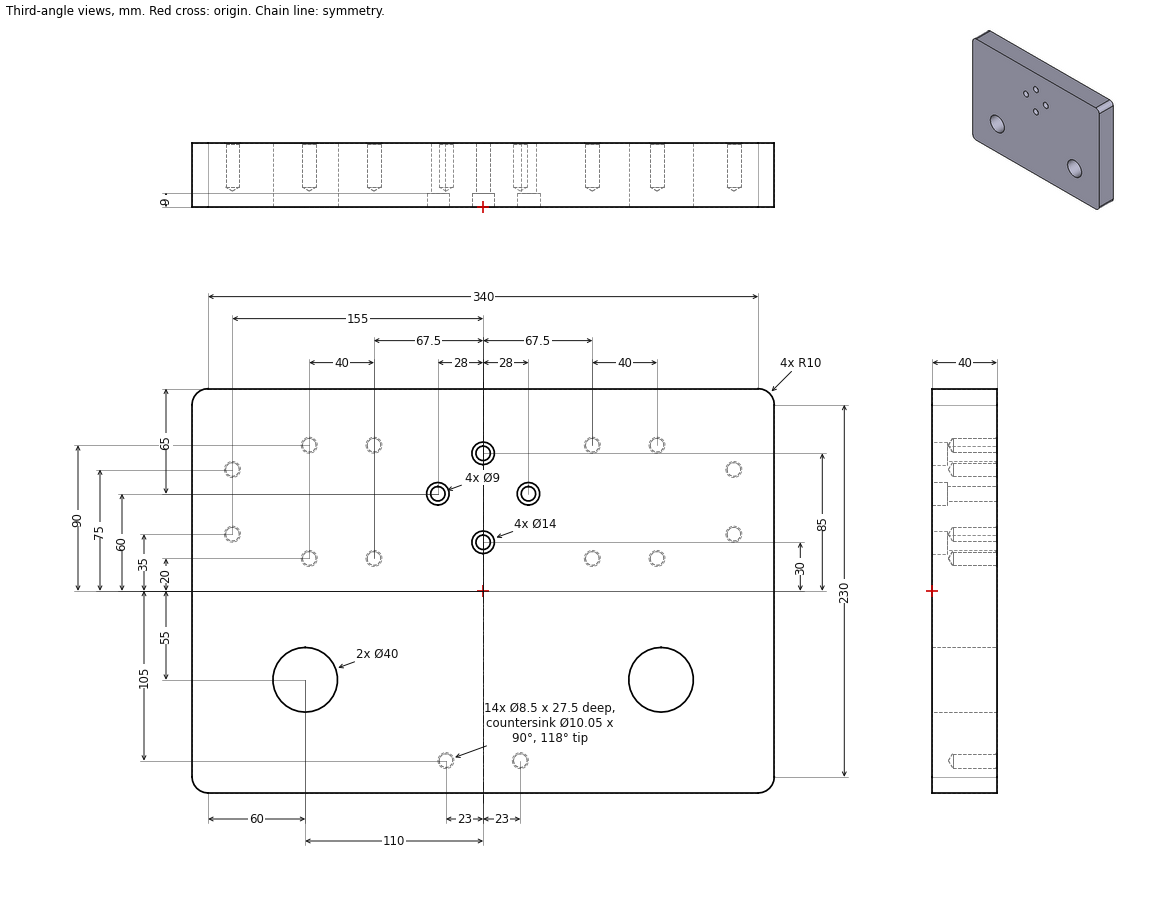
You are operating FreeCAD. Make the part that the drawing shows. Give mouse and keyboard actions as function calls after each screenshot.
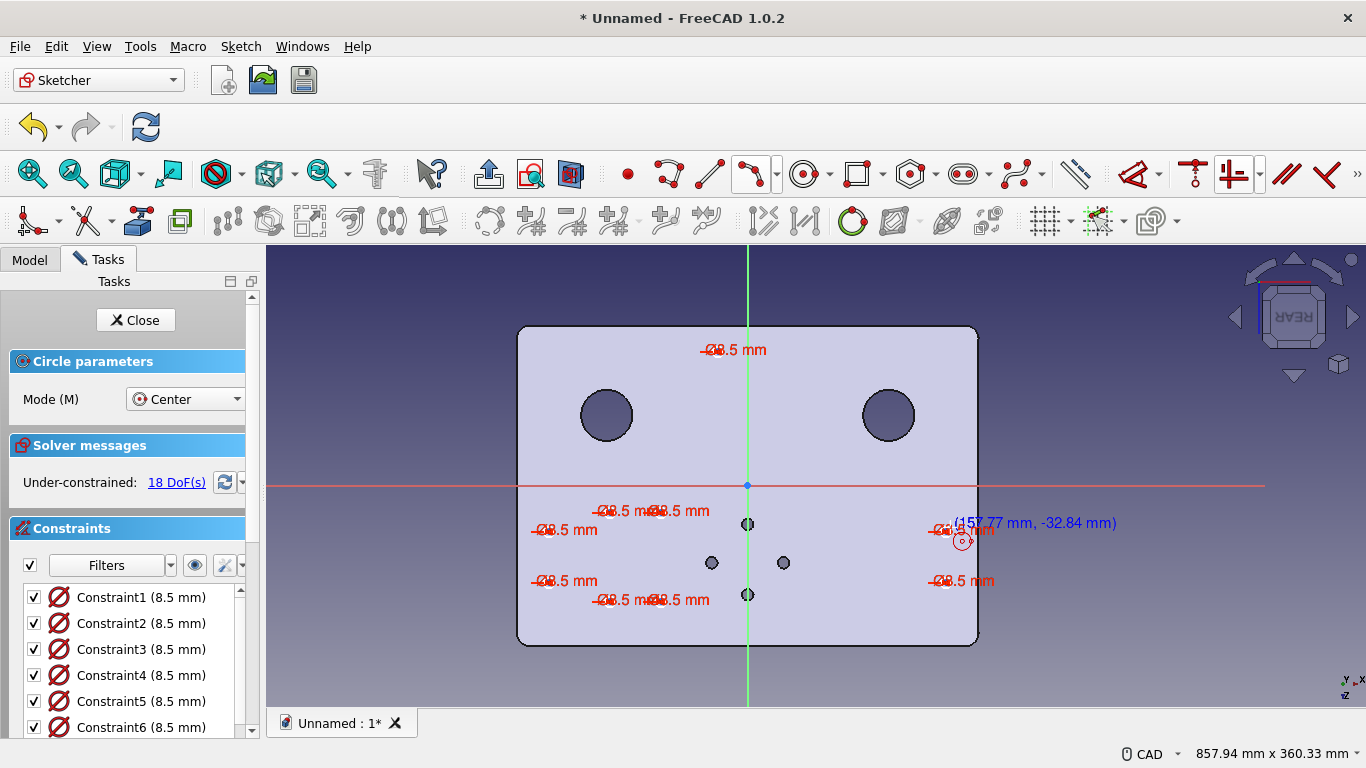
scroll(834, 601, up, 8)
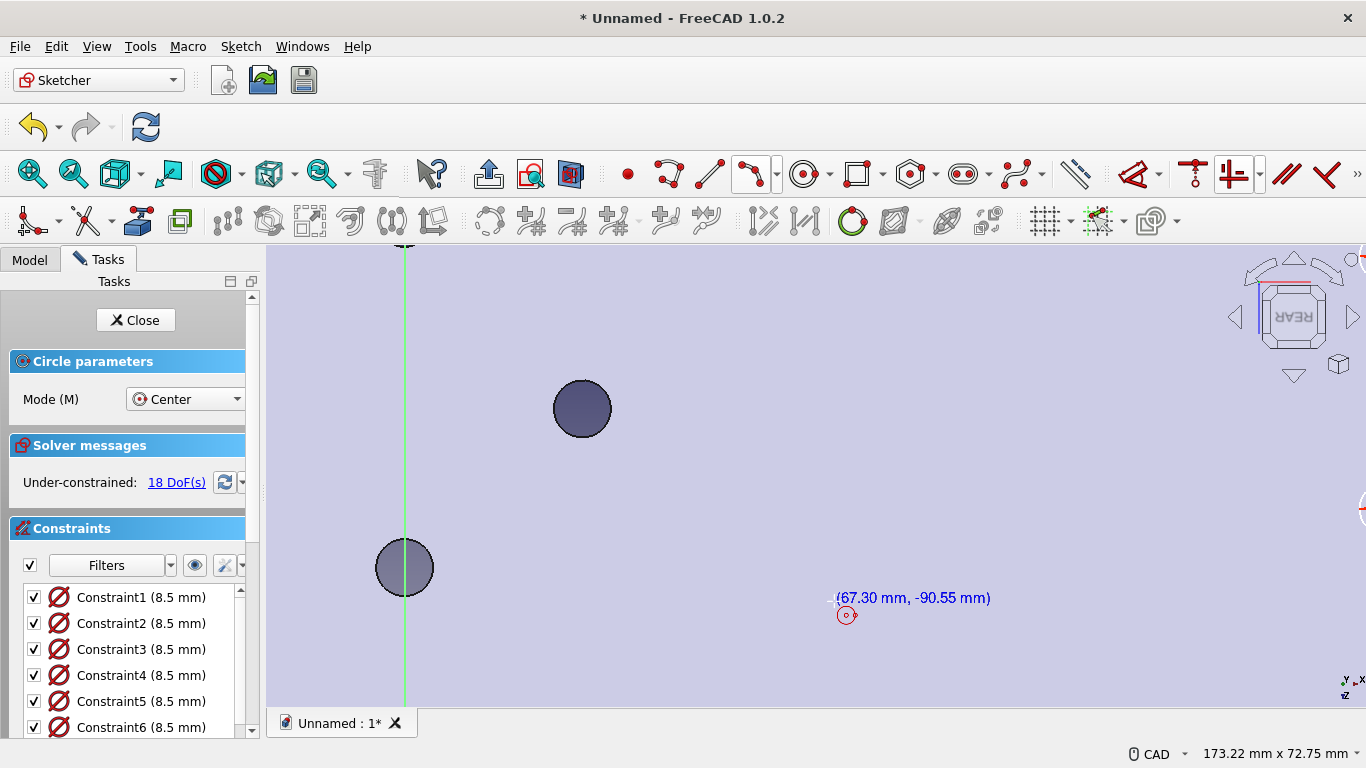
scroll(834, 601, down, 8)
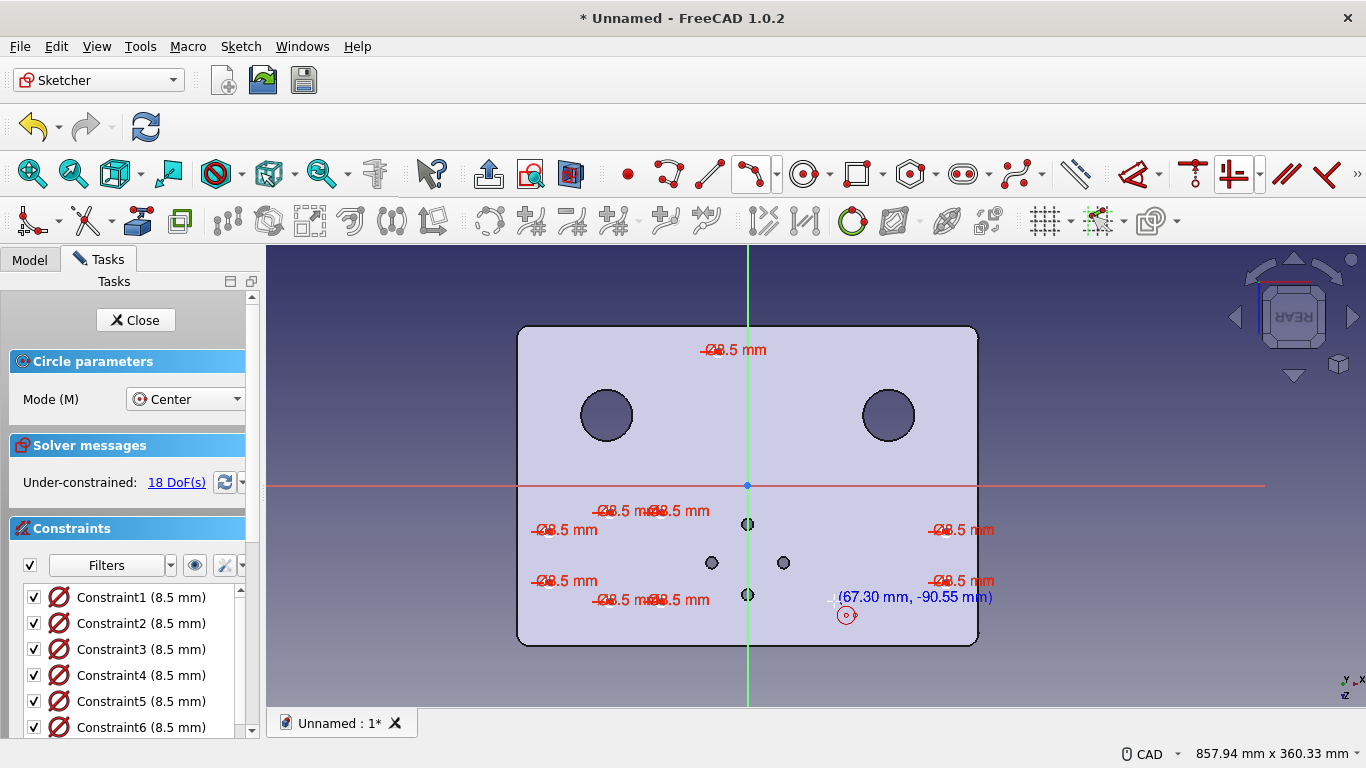
click(834, 601)
move(838, 597)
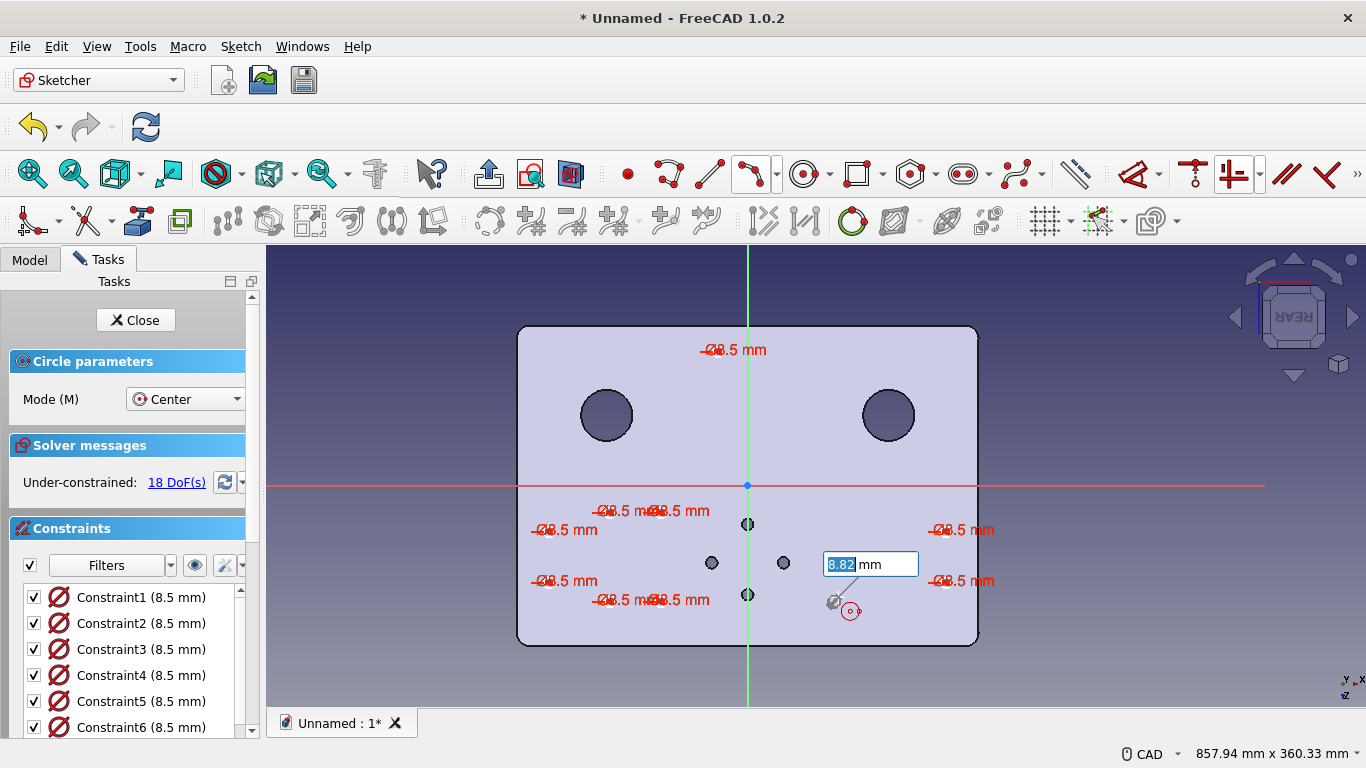
text(8.5)
key(Return)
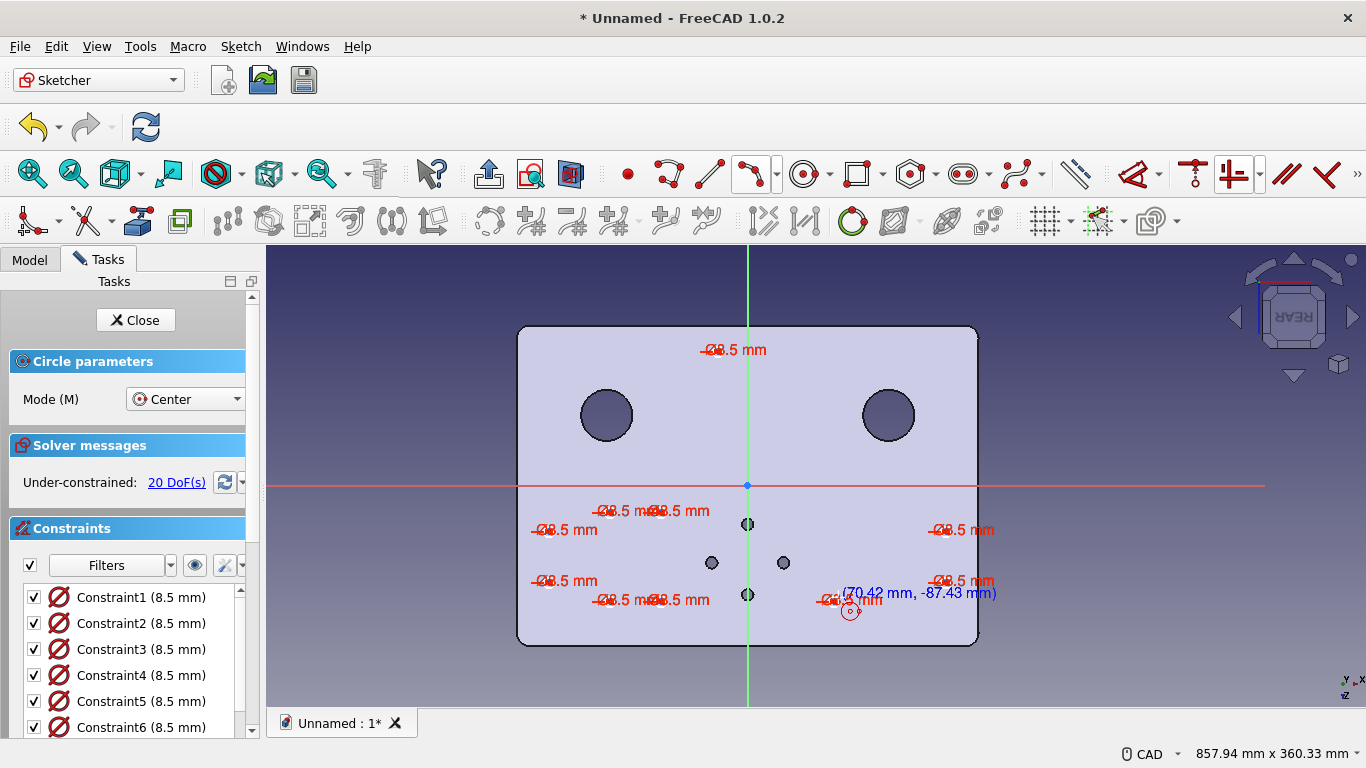
scroll(886, 601, up, 8)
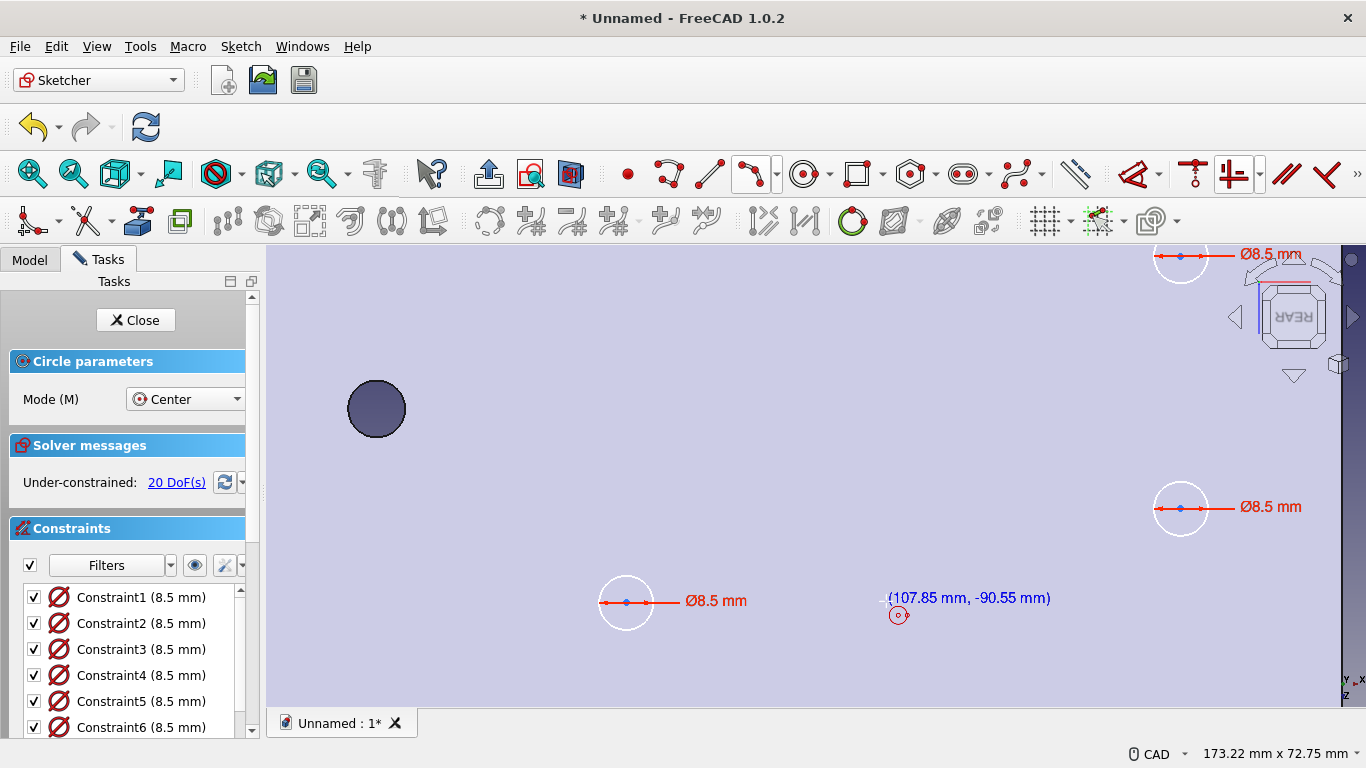
scroll(886, 601, down, 8)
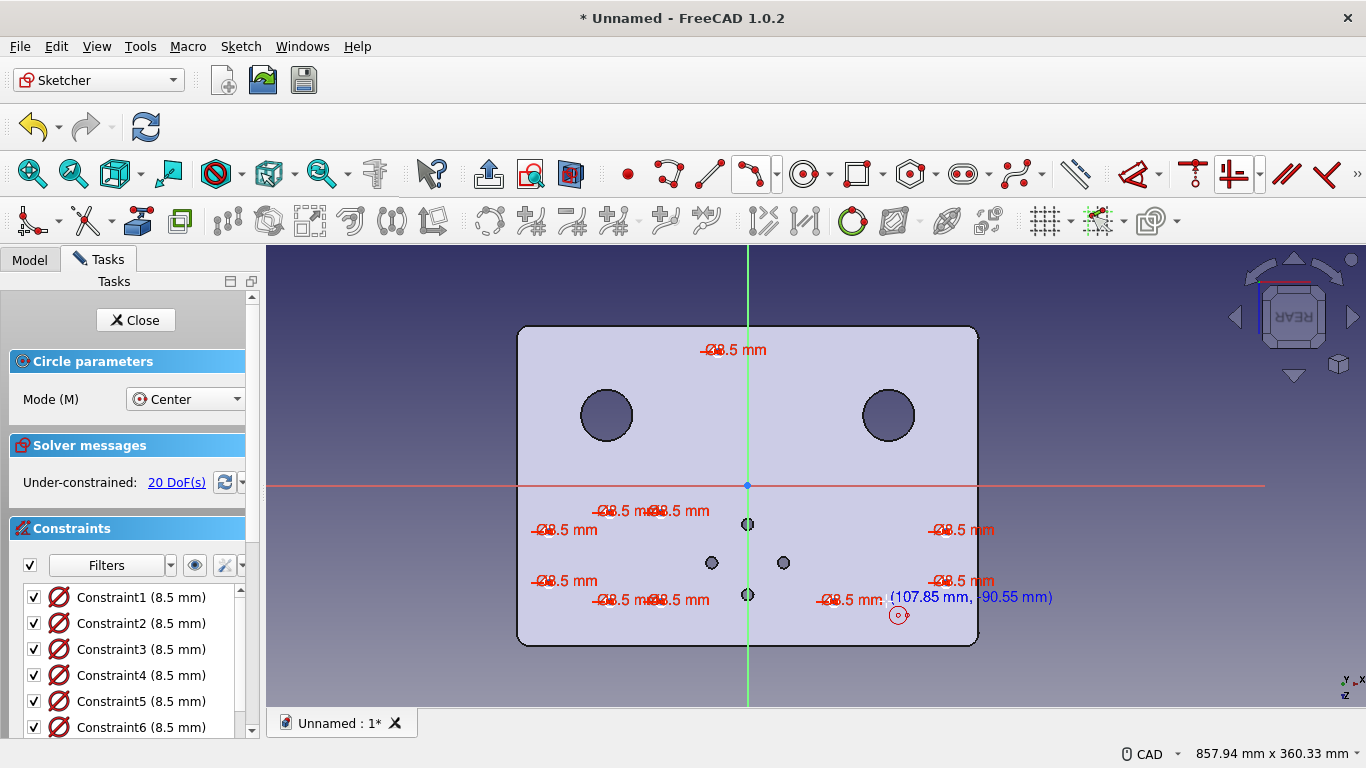
click(886, 601)
move(889, 597)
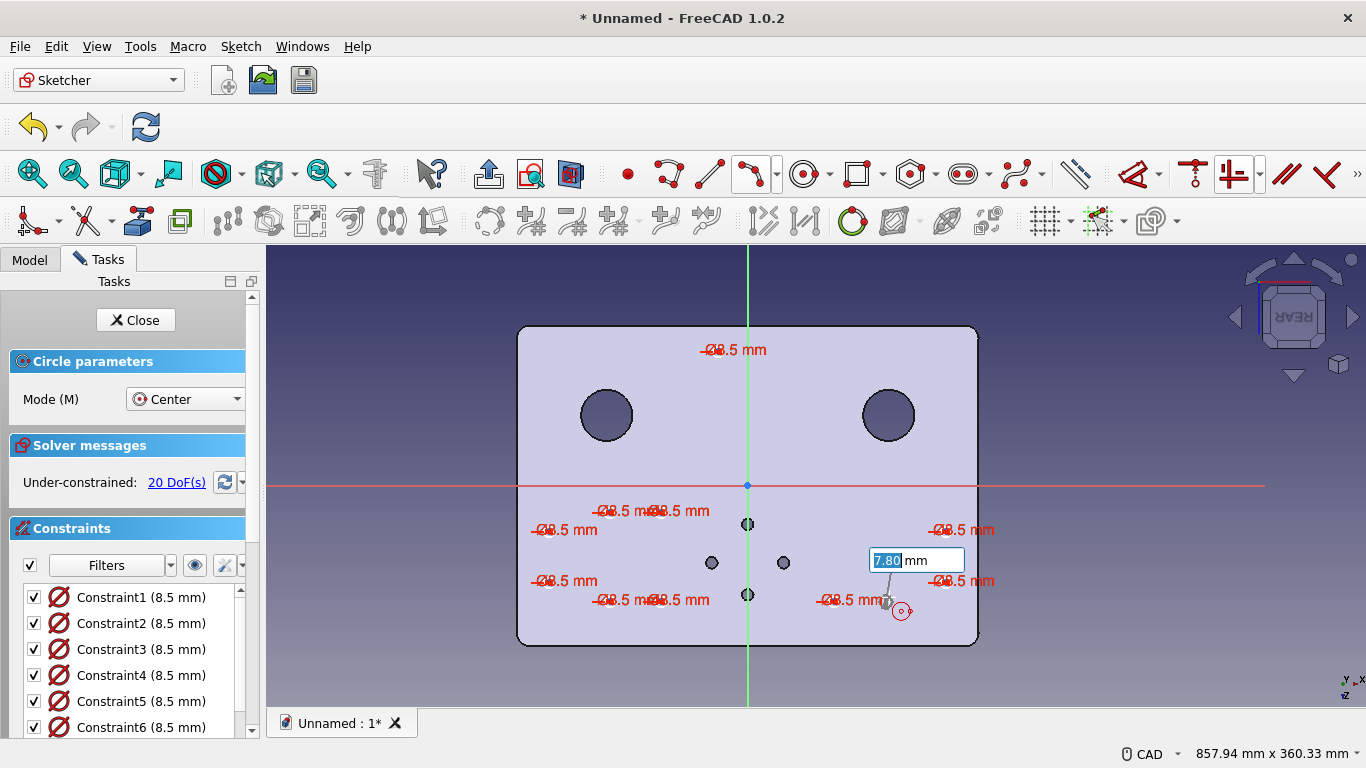
text(8.5)
key(Return)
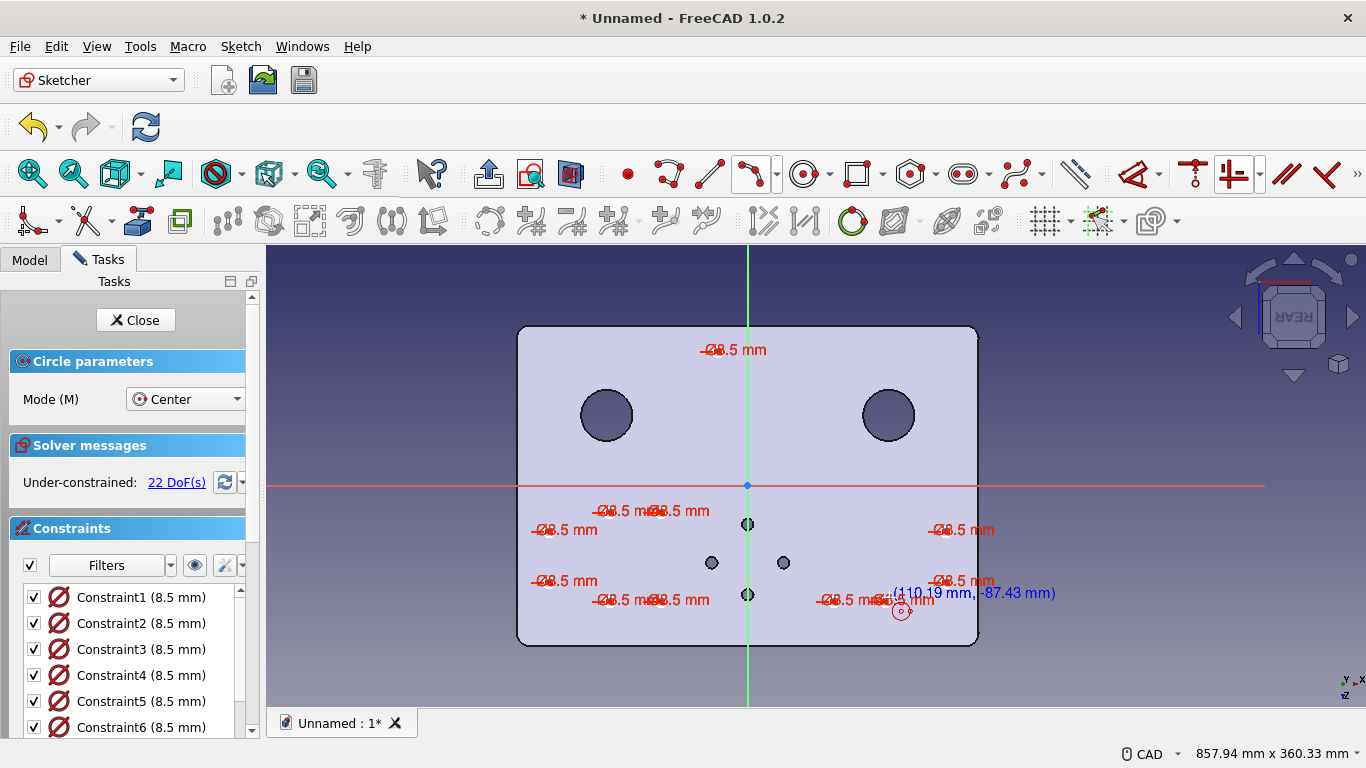
scroll(834, 512, up, 8)